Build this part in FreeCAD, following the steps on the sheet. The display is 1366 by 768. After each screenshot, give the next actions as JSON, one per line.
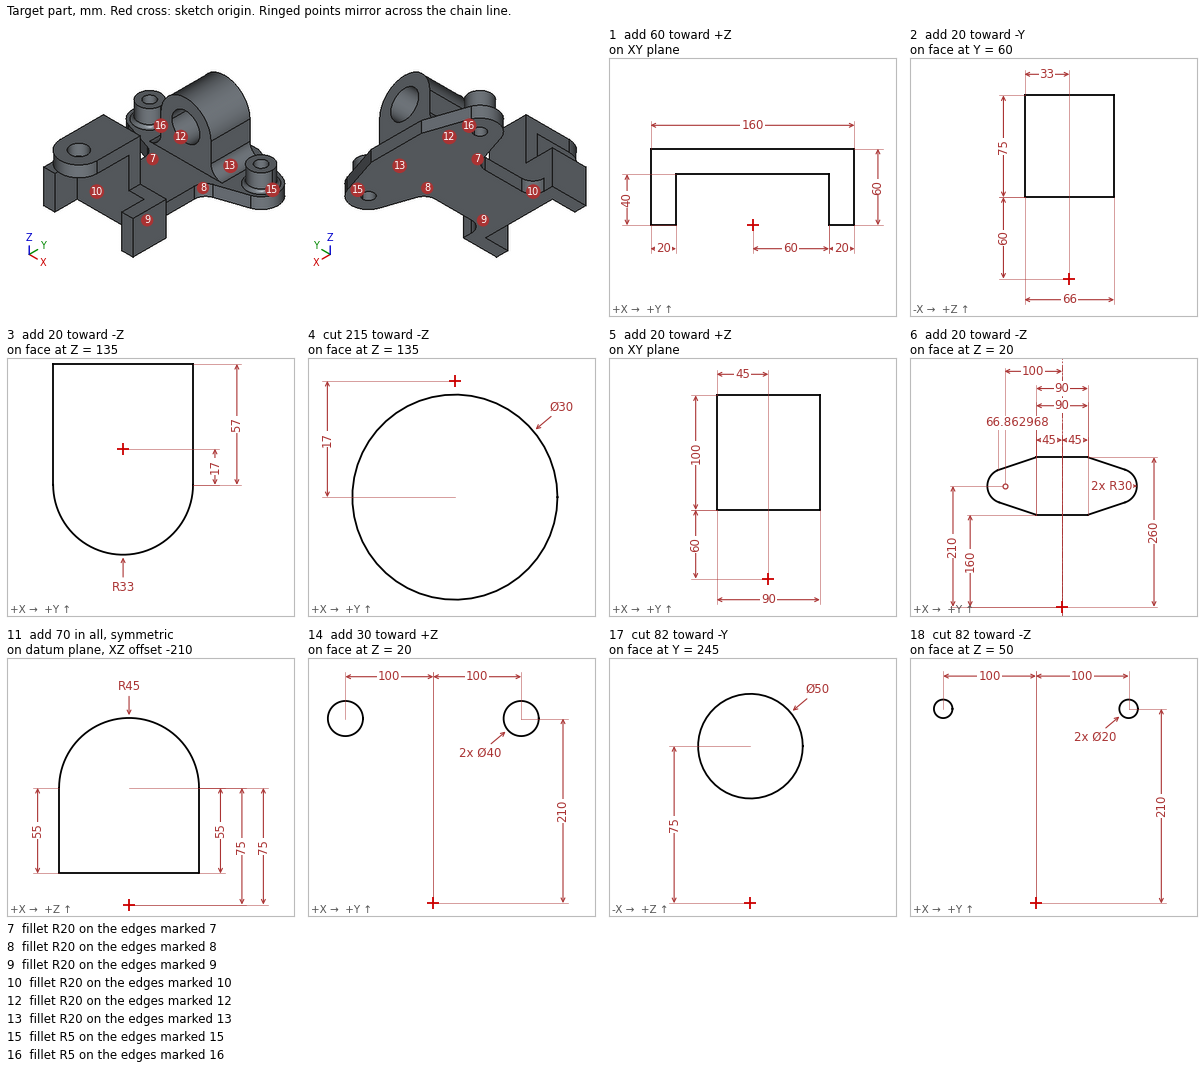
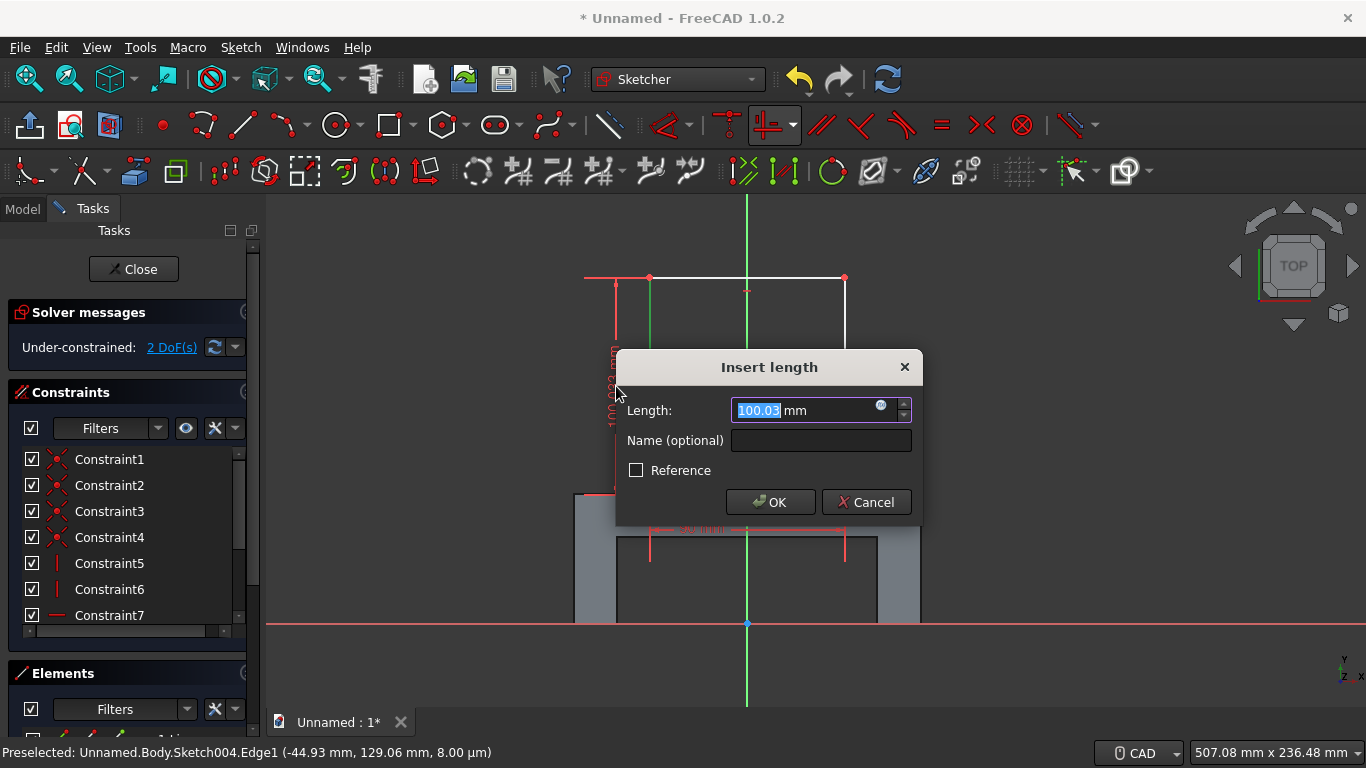
{"action": "type", "text": "100"}
{"action": "key", "text": "Return"}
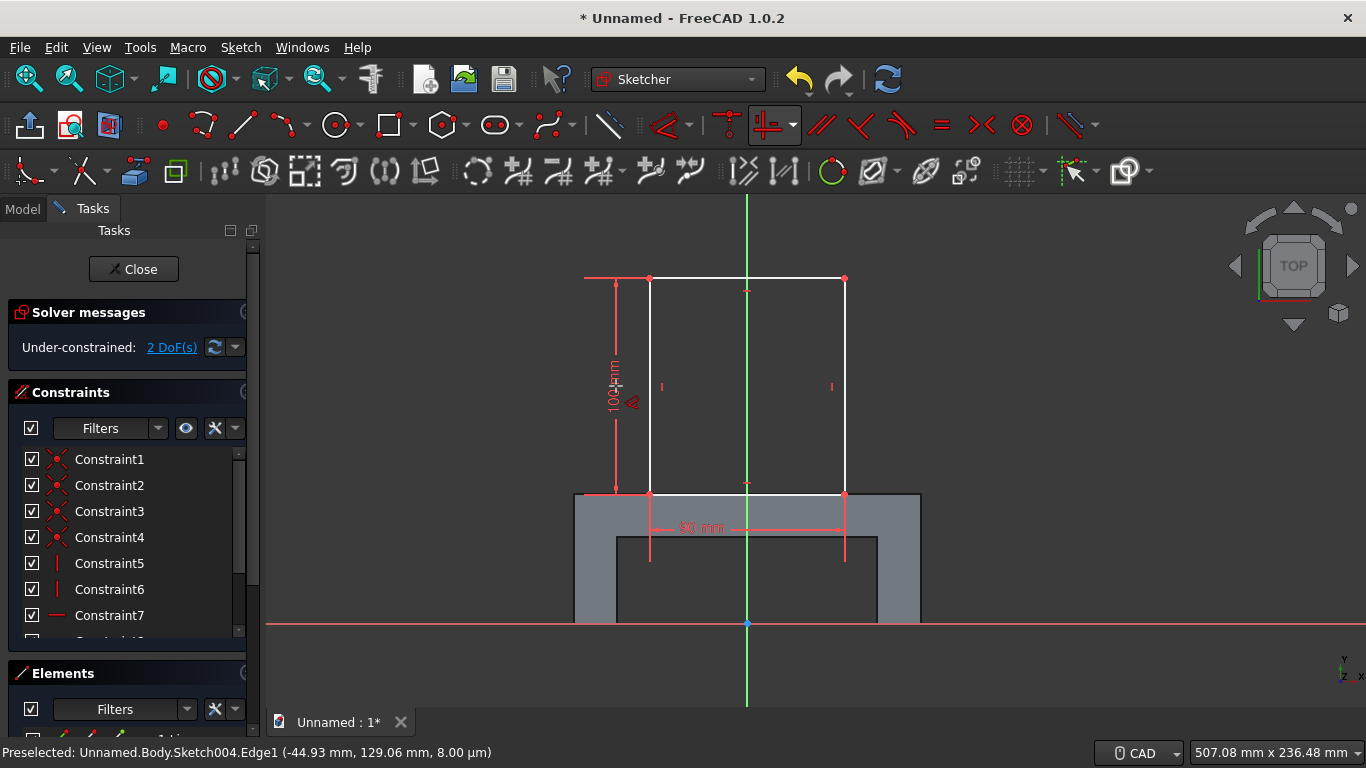
{"action": "left_click", "coordinate": [650, 278]}
{"action": "left_click", "coordinate": [698, 658]}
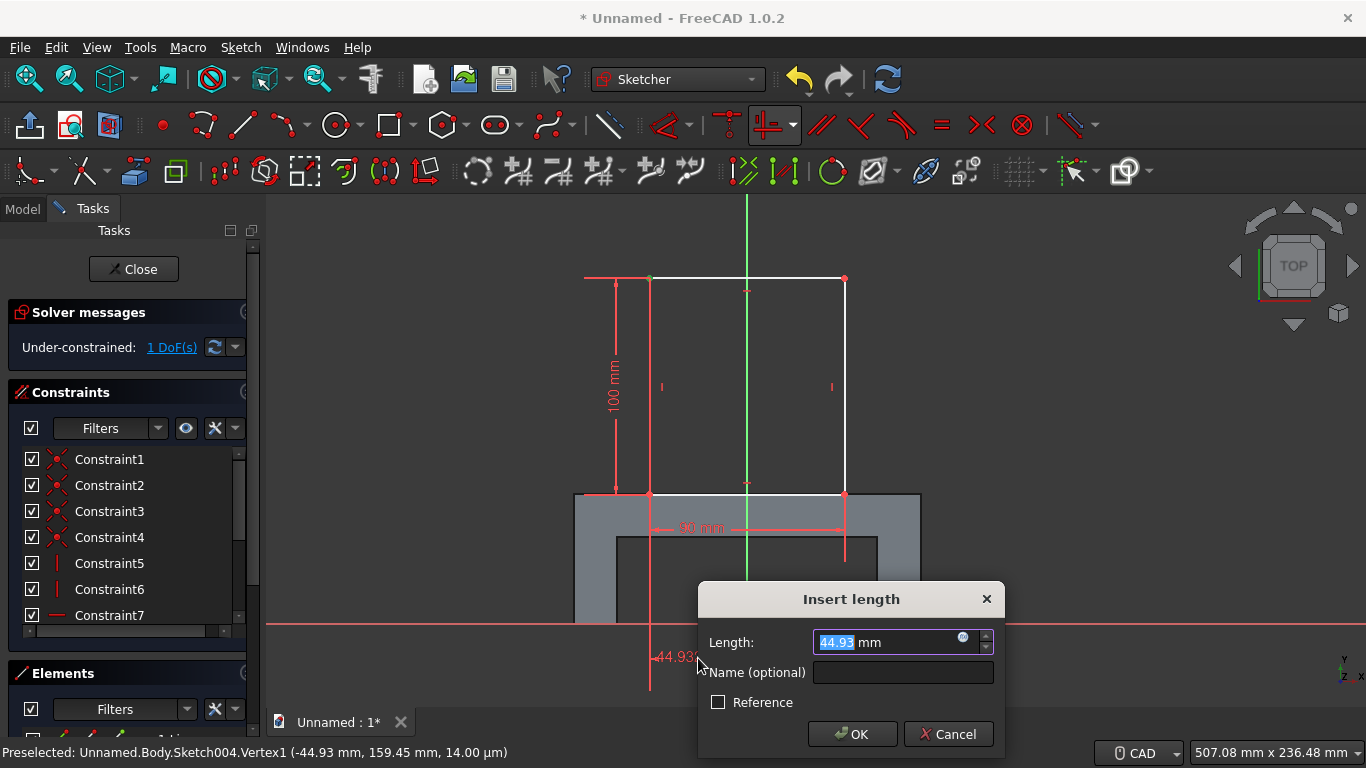
{"action": "type", "text": "45"}
{"action": "key", "text": "Return"}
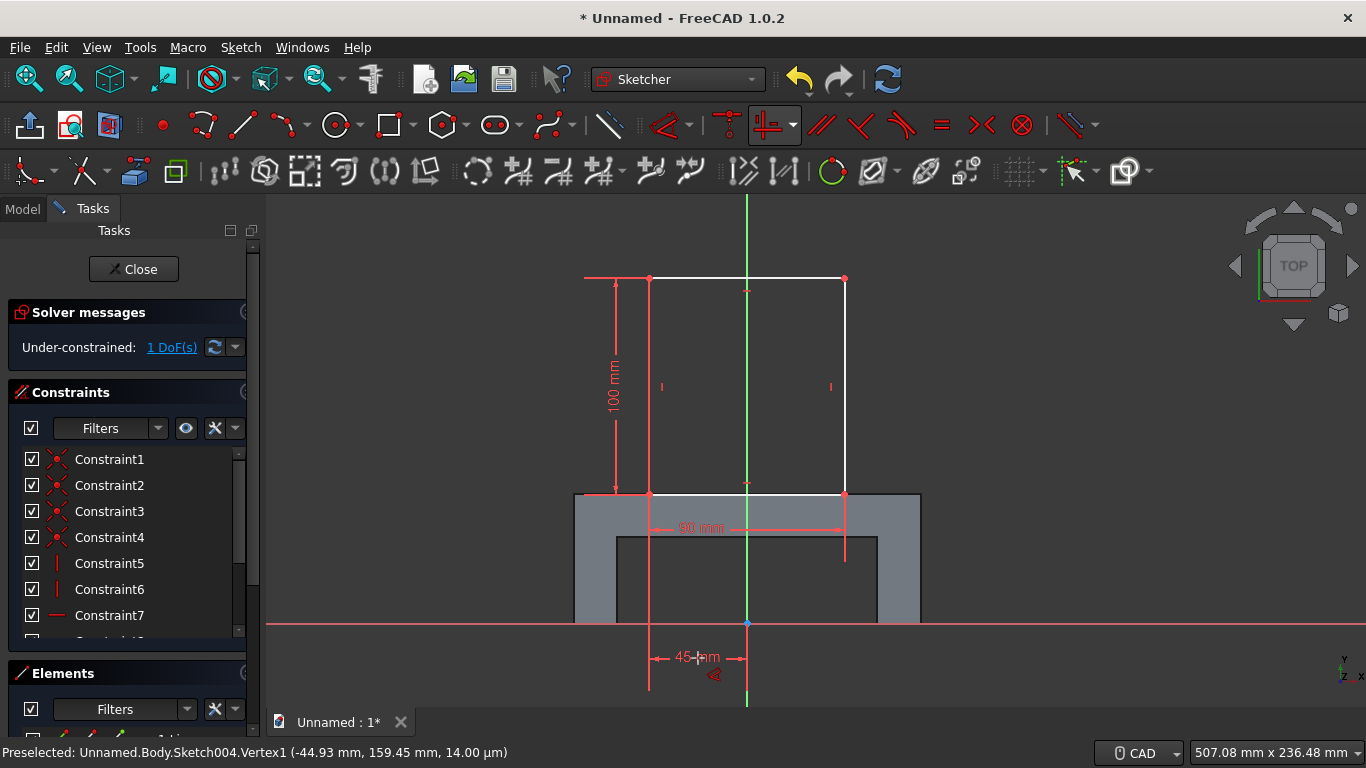
{"action": "left_click", "coordinate": [649, 495]}
{"action": "left_click", "coordinate": [615, 559]}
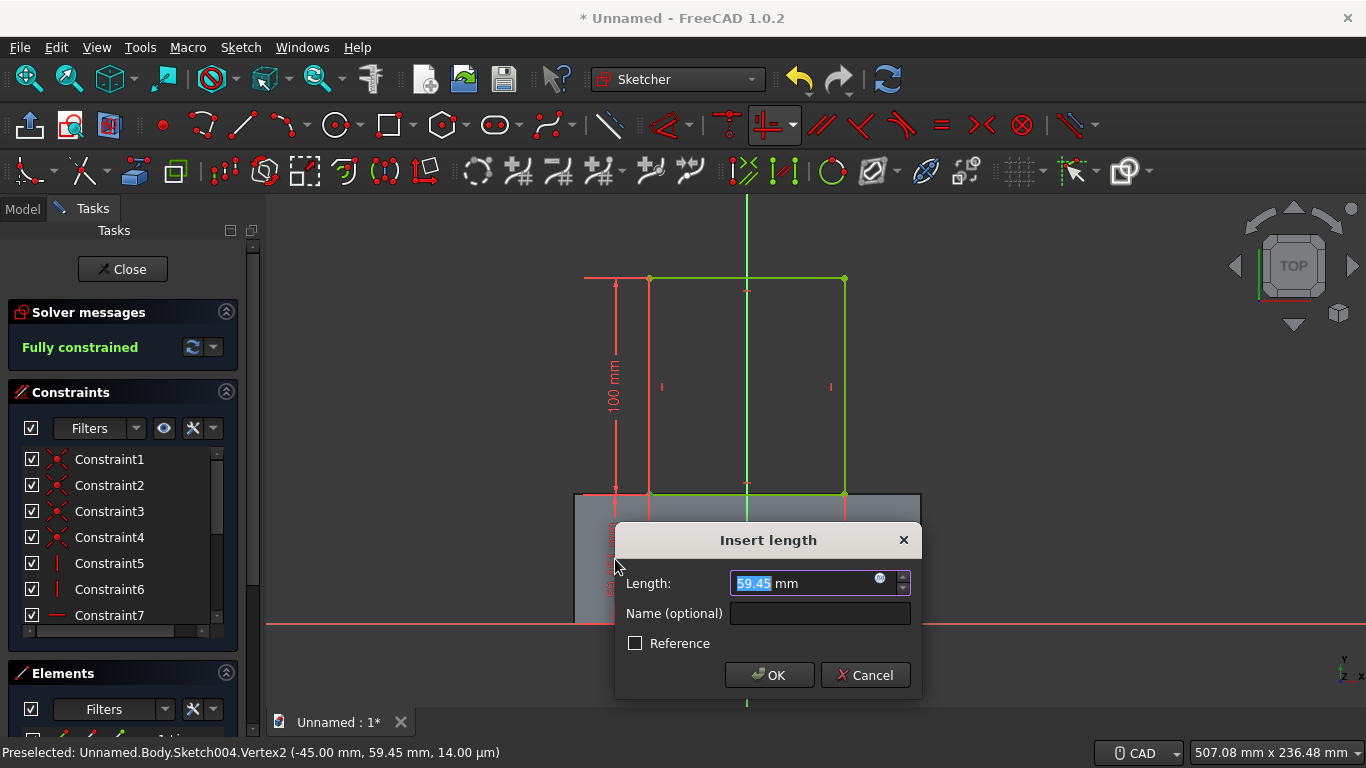
{"action": "type", "text": "60"}
{"action": "key", "text": "Return"}
{"action": "key", "text": "Escape"}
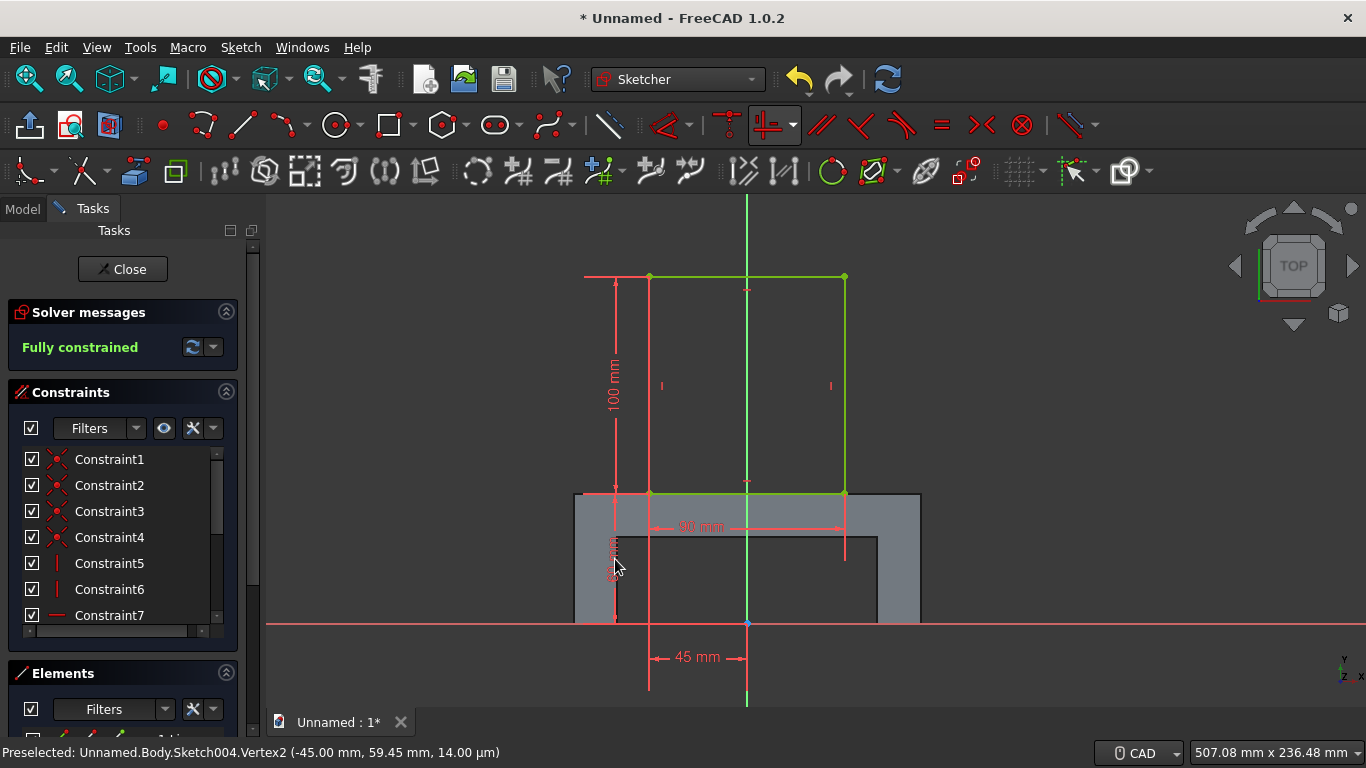
{"action": "left_click", "coordinate": [123, 269]}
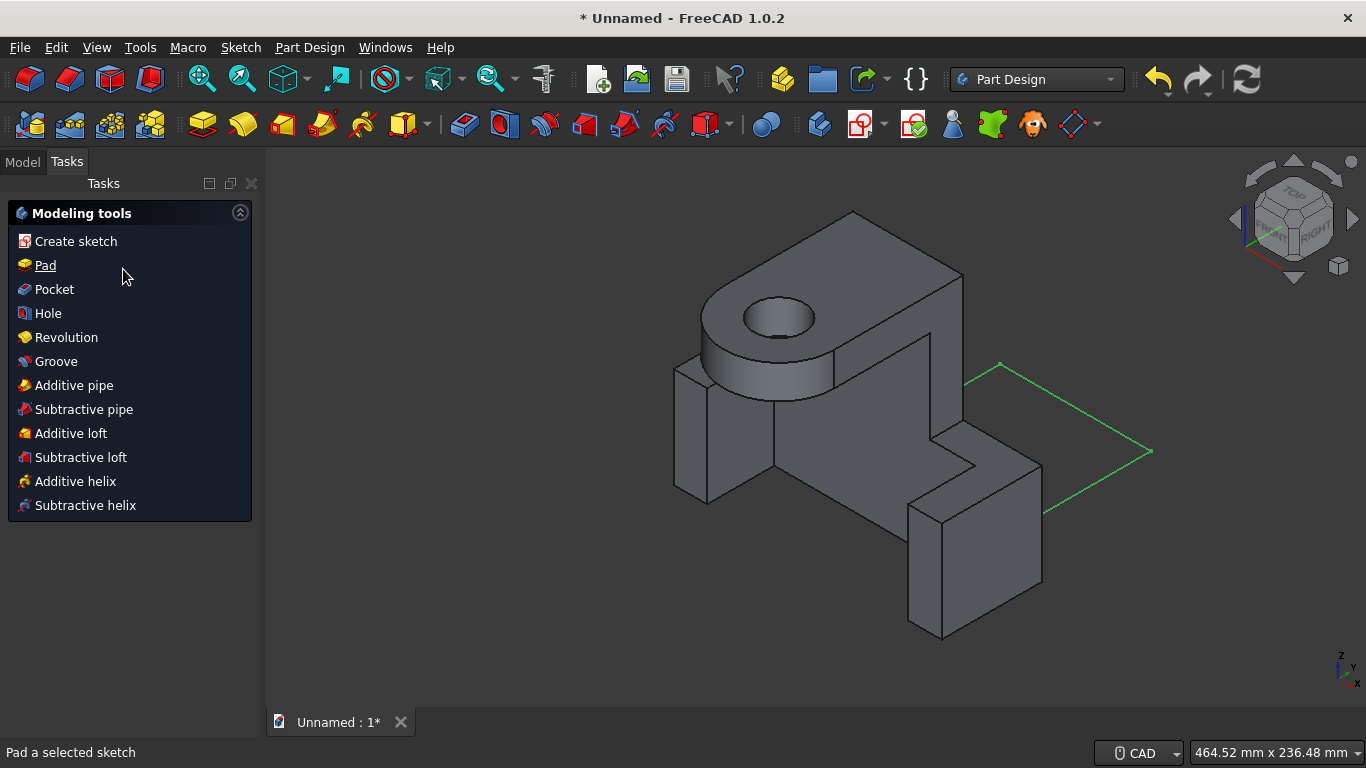
{"action": "left_click", "coordinate": [204, 124]}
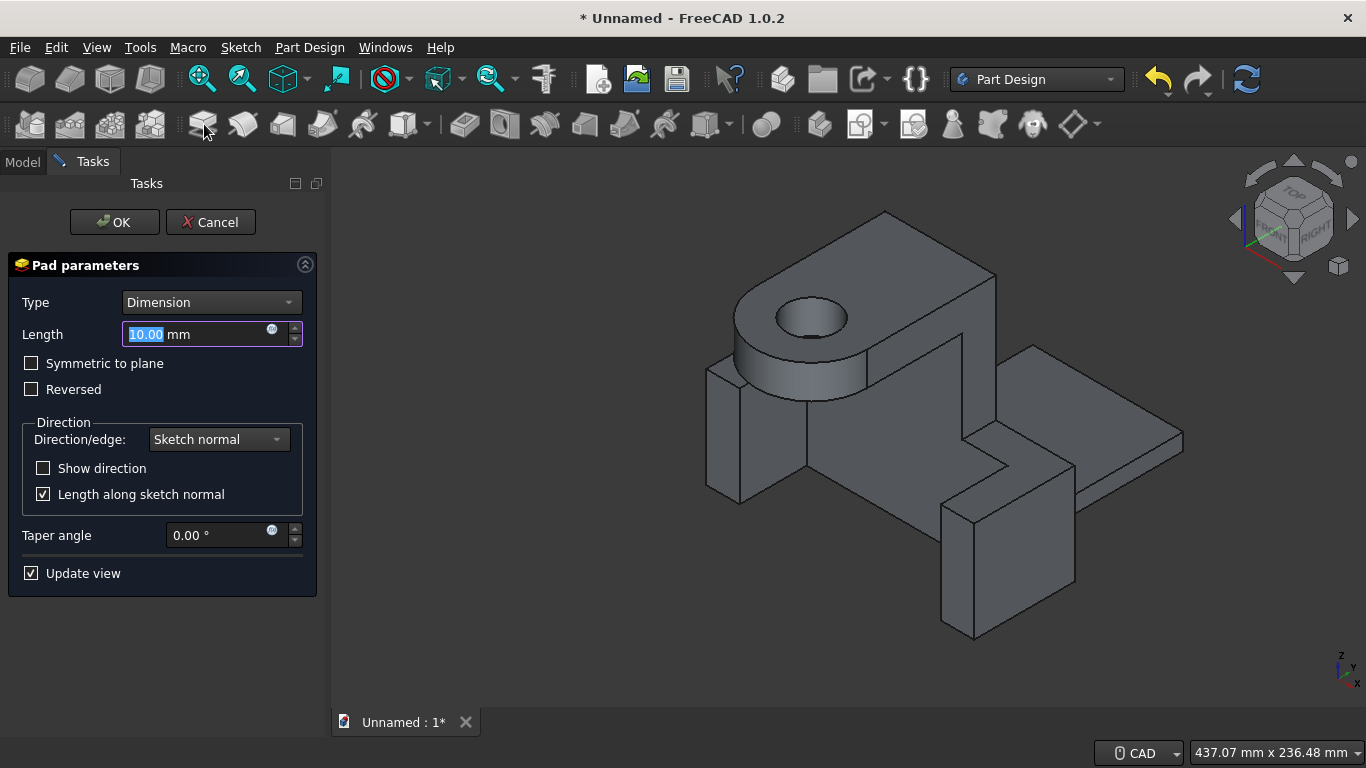
{"action": "type", "text": "20"}
{"action": "key", "text": "Tab"}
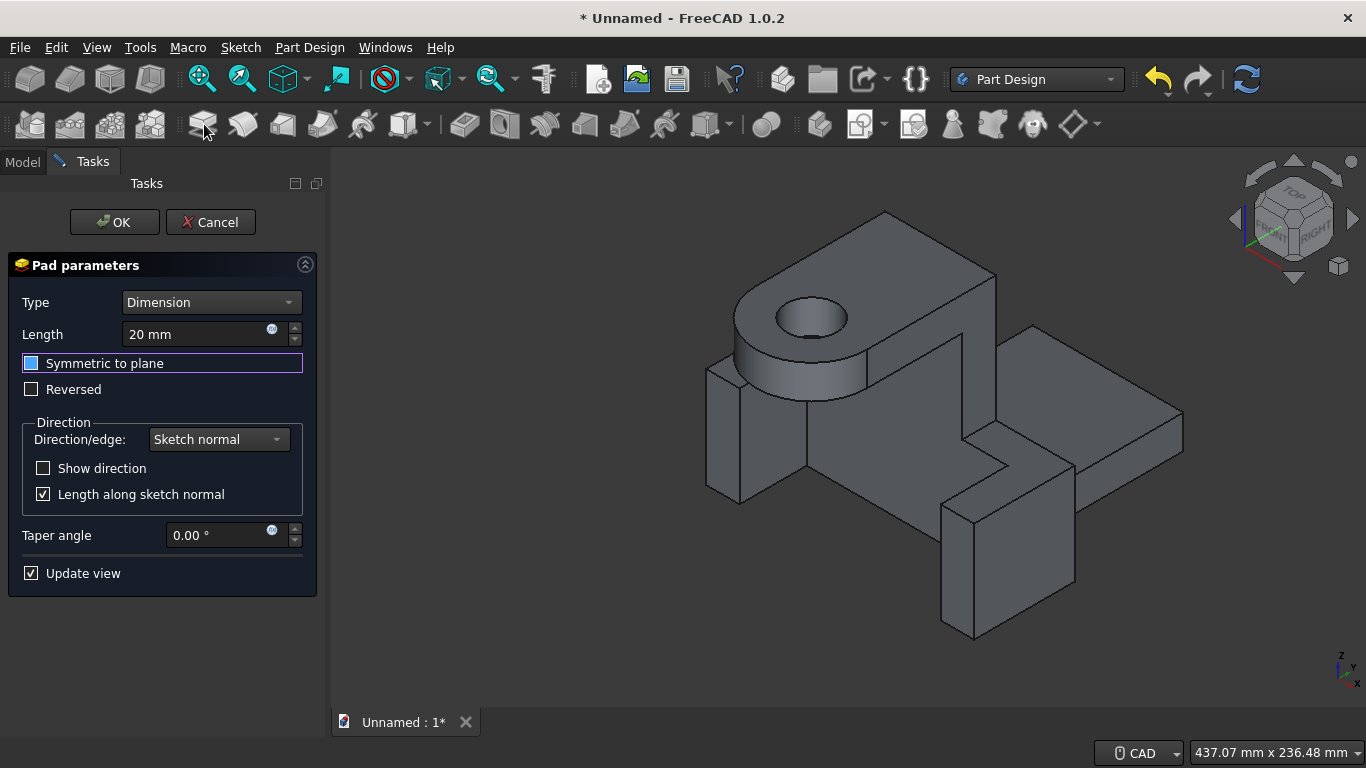
{"action": "left_click", "coordinate": [115, 222]}